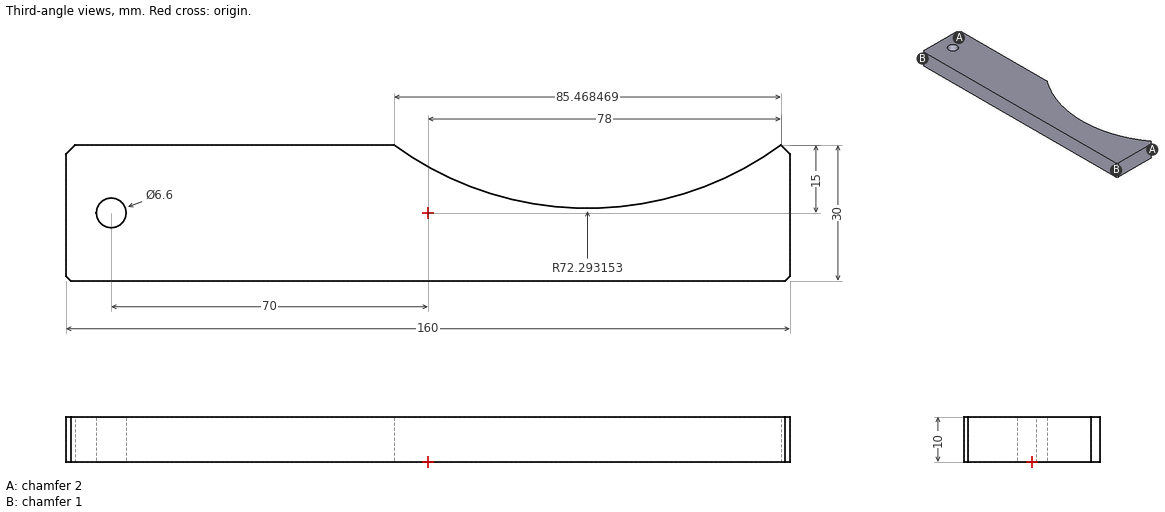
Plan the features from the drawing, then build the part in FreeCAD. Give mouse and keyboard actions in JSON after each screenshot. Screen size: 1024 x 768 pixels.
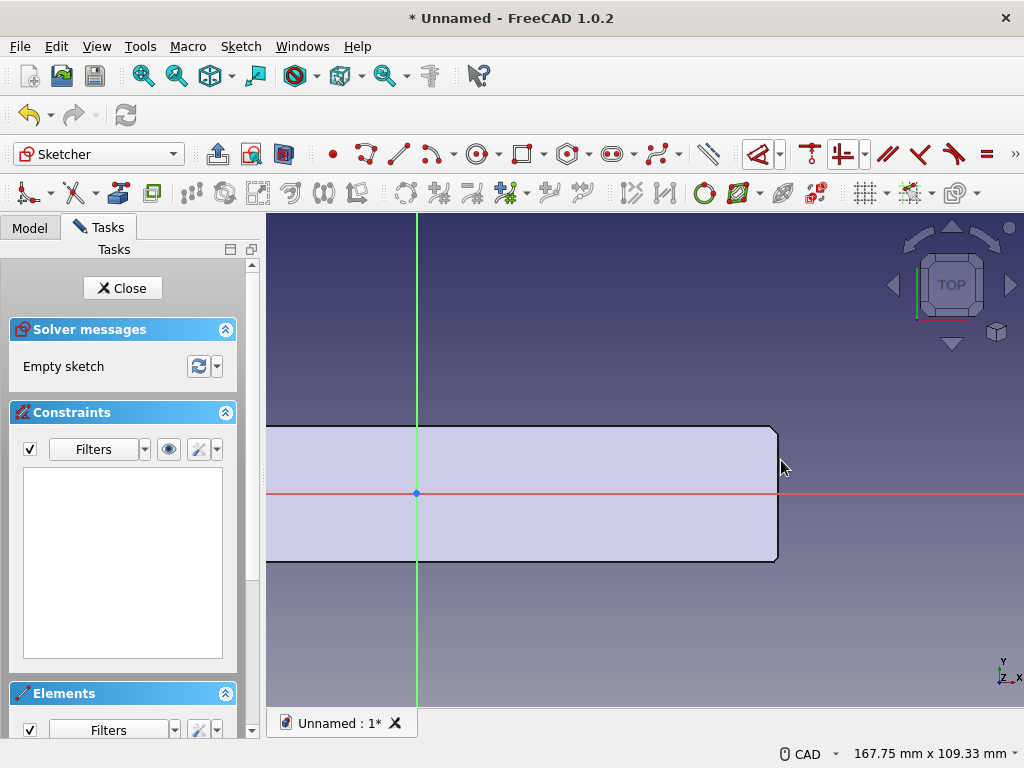
{"action": "left_click", "coordinate": [399, 154]}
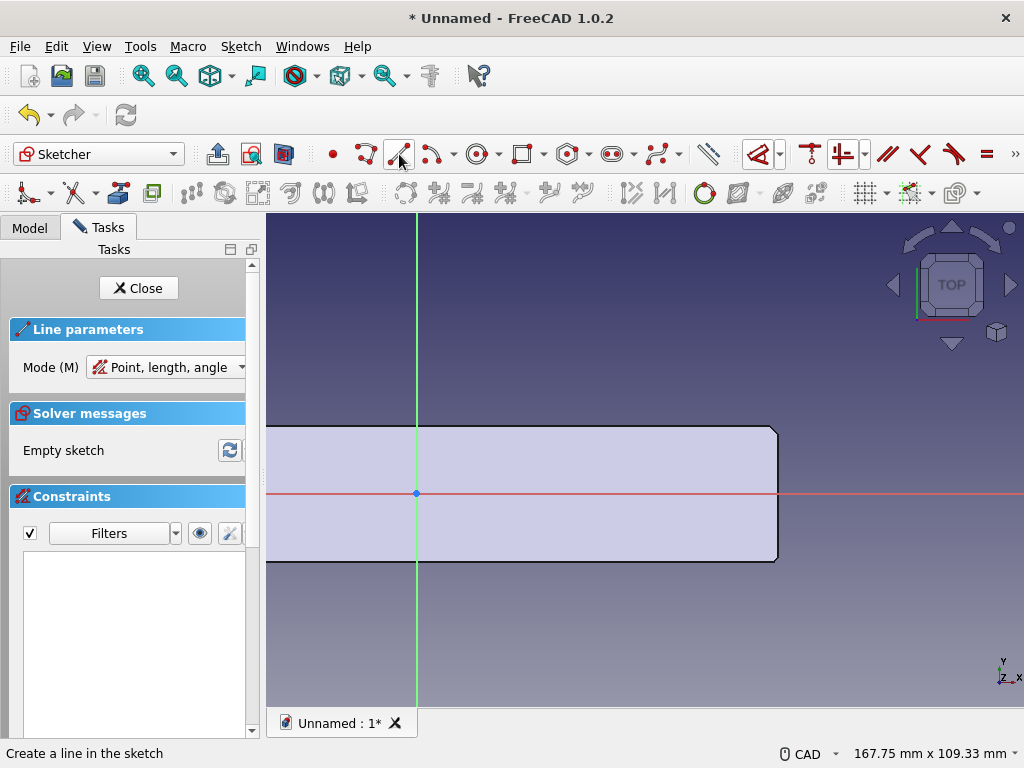
{"action": "left_click", "coordinate": [769, 426]}
{"action": "left_click", "coordinate": [383, 426]}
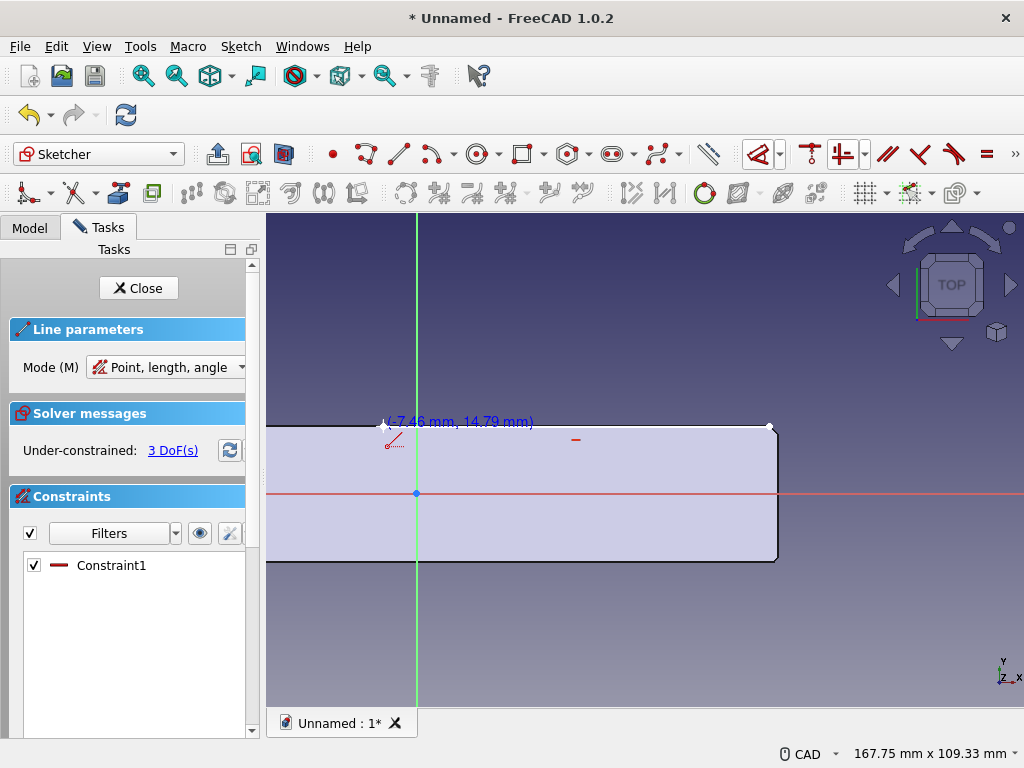
{"action": "key", "text": "g 3 a"}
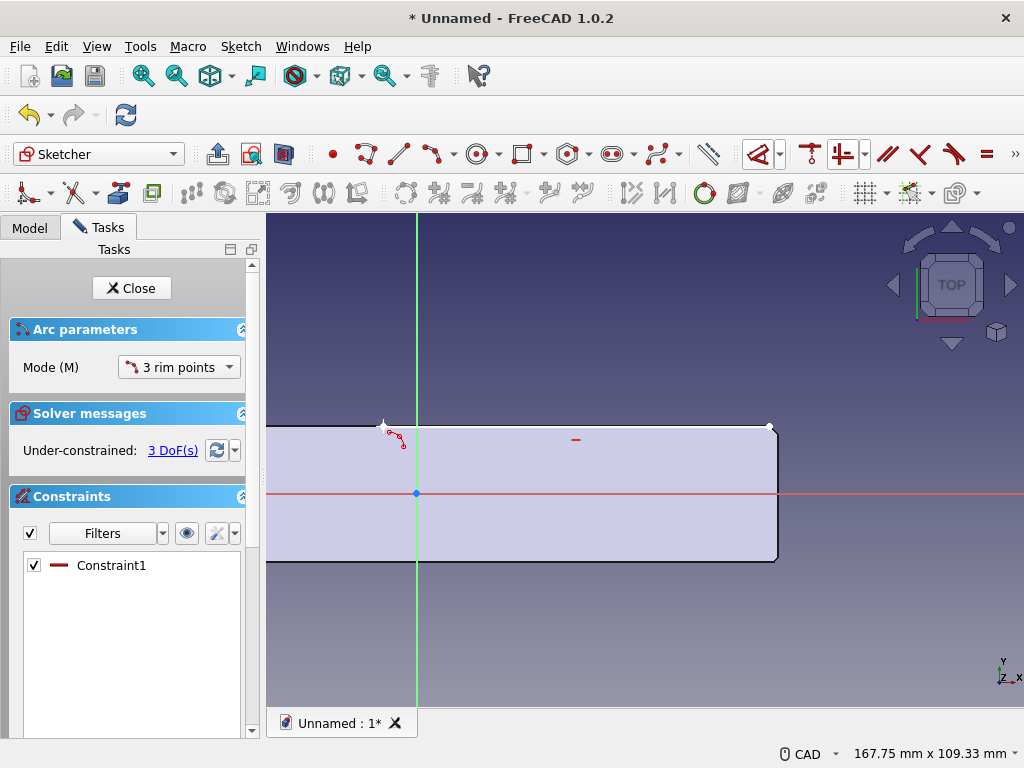
{"action": "left_click", "coordinate": [383, 427]}
{"action": "left_click", "coordinate": [769, 427]}
{"action": "left_click", "coordinate": [494, 479]}
{"action": "key", "text": "Escape"}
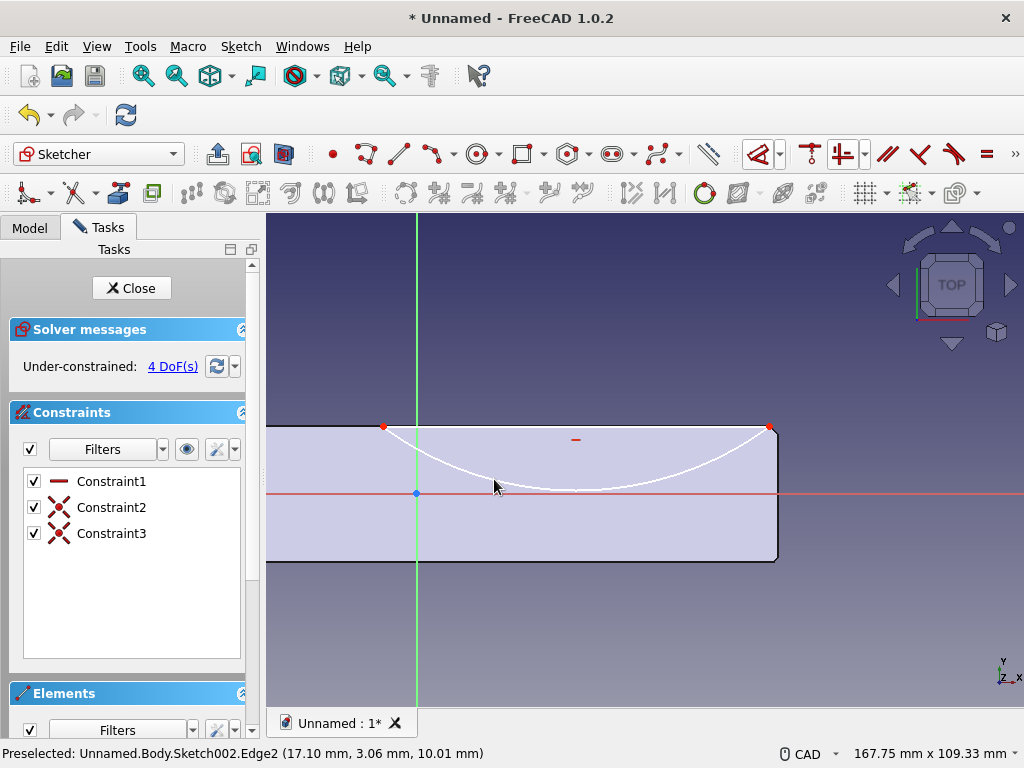
{"action": "left_click", "coordinate": [758, 154]}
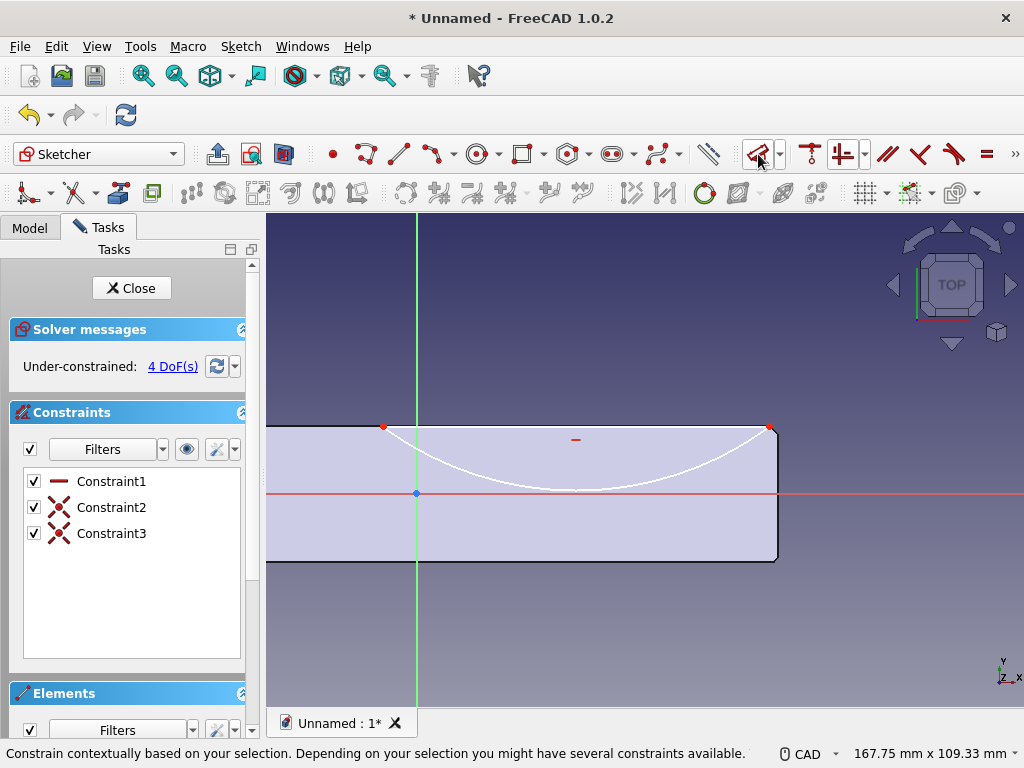
{"action": "left_click", "coordinate": [494, 480]}
{"action": "left_click", "coordinate": [486, 511]}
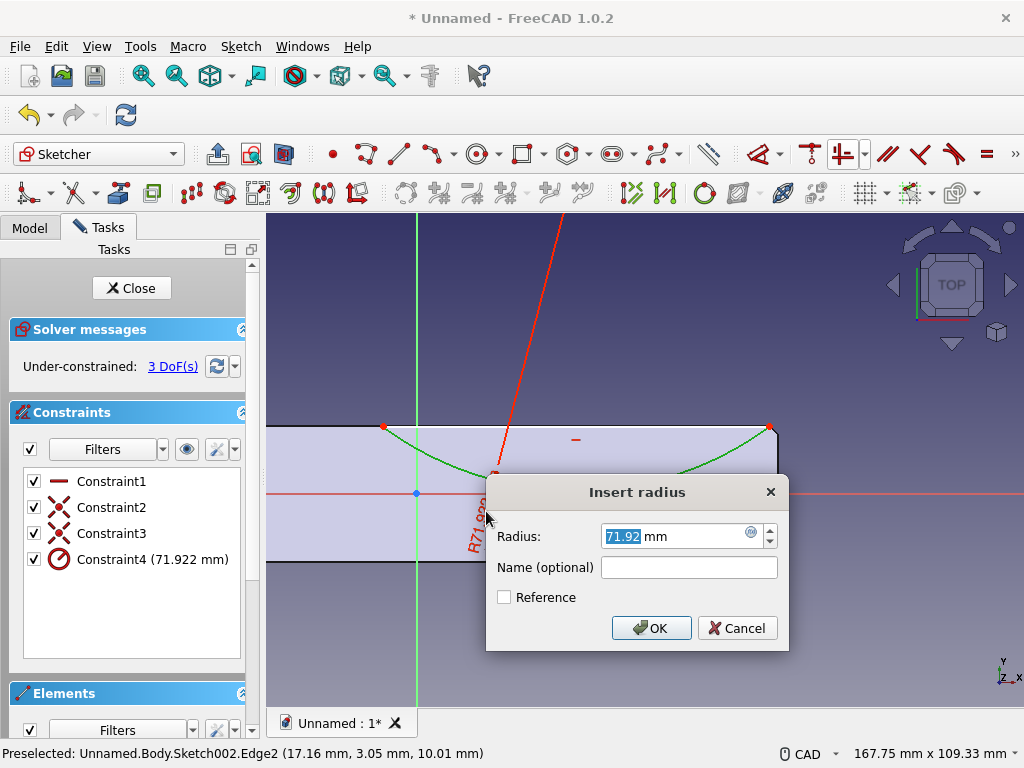
{"action": "type", "text": "72.293153"}
{"action": "key", "text": "Return"}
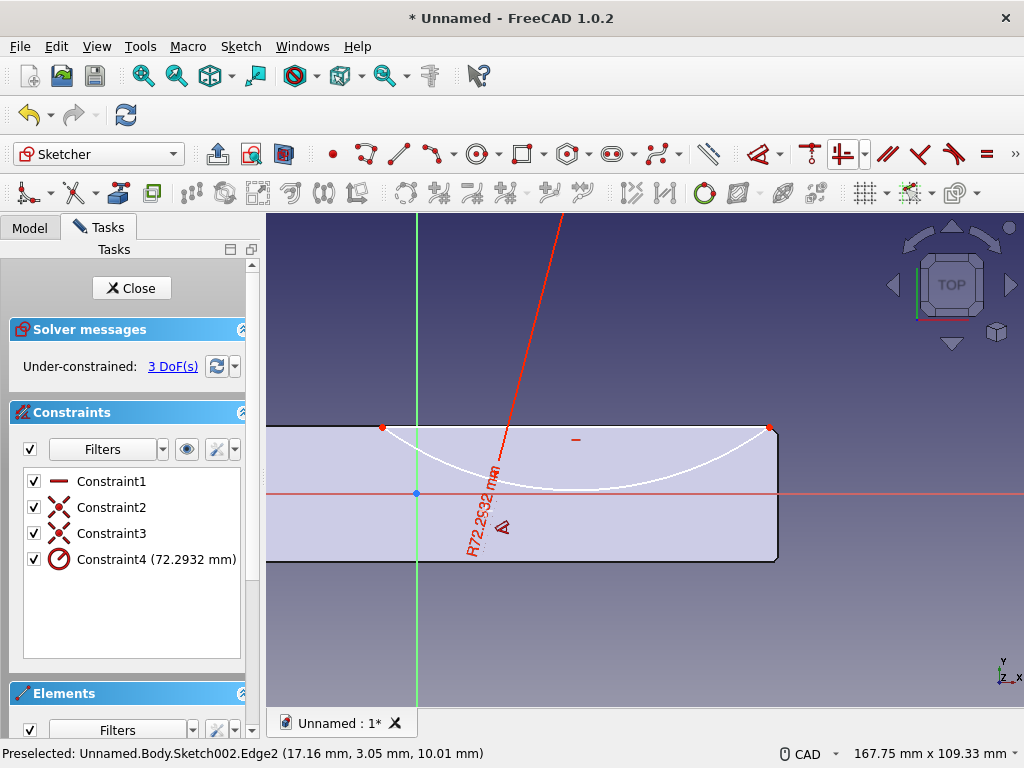
{"action": "left_click", "coordinate": [769, 427]}
{"action": "left_click", "coordinate": [593, 528]}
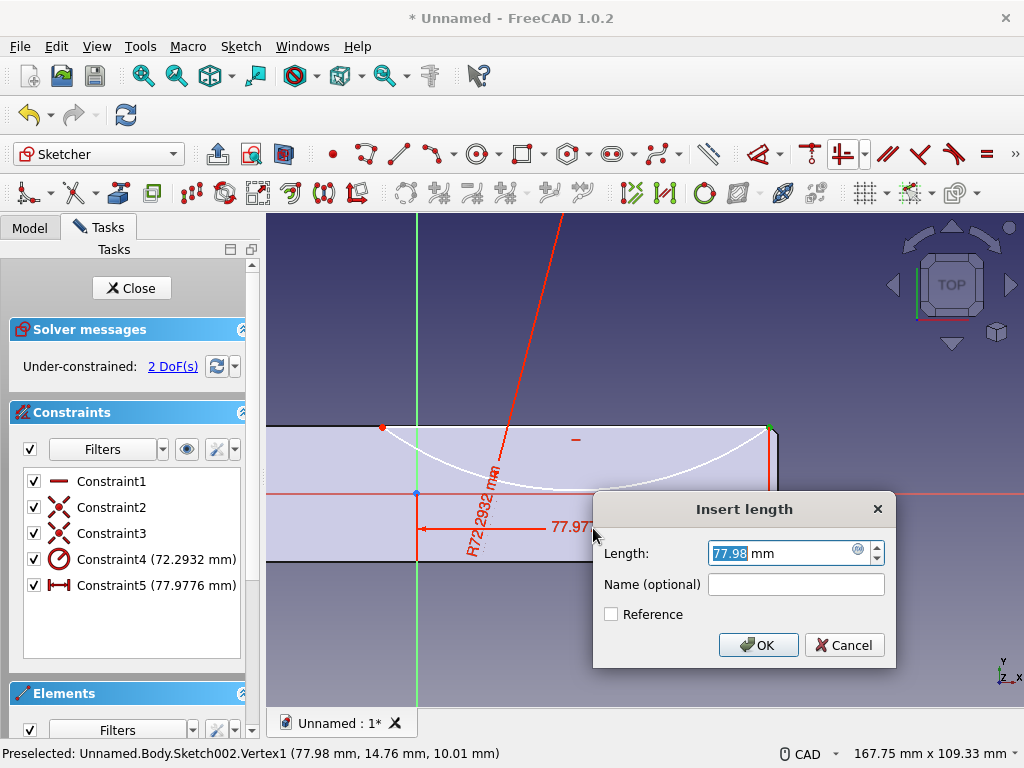
{"action": "type", "text": "78"}
{"action": "key", "text": "Return"}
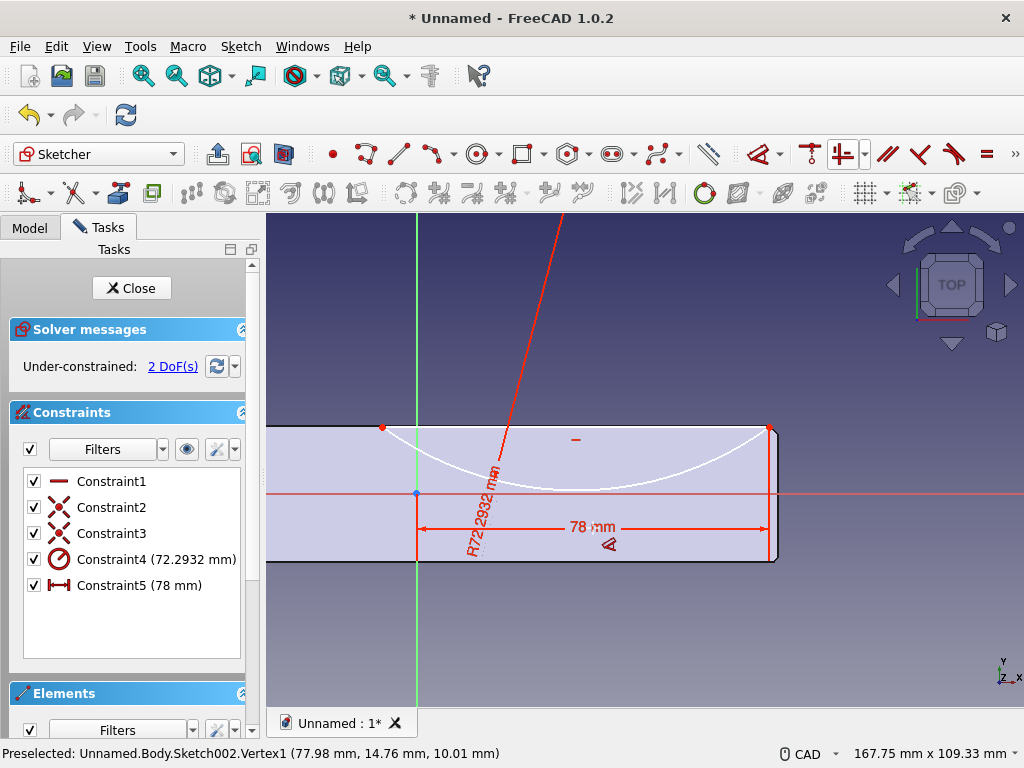
{"action": "left_click", "coordinate": [769, 427]}
{"action": "left_click", "coordinate": [803, 461]}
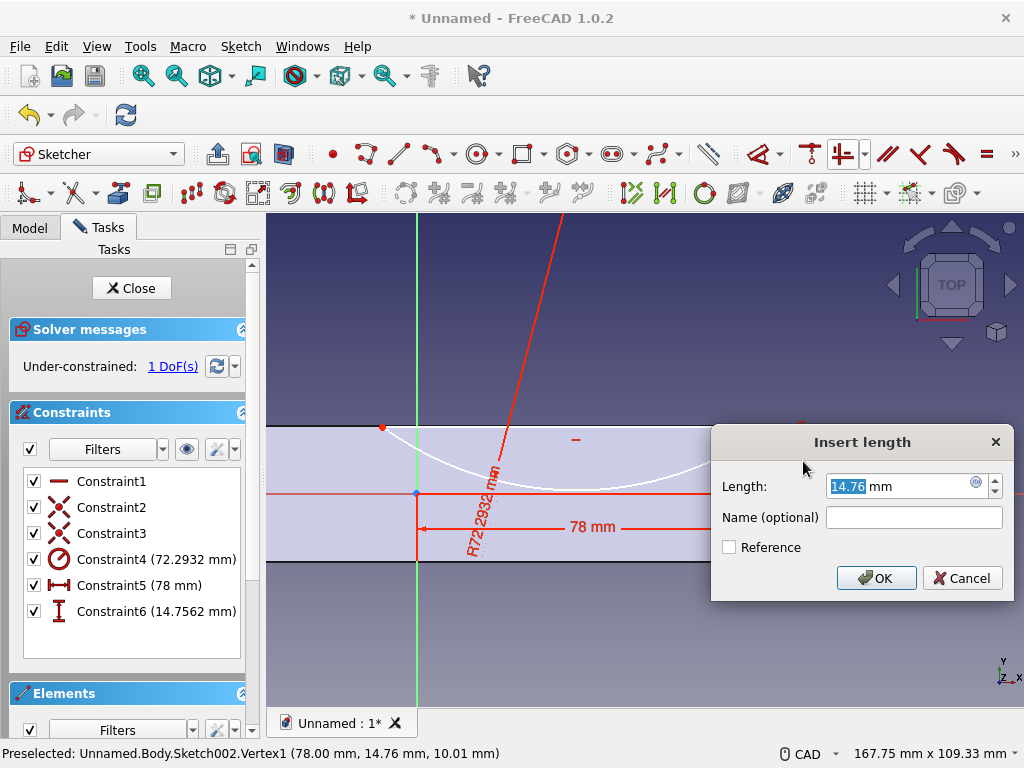
{"action": "type", "text": "15"}
{"action": "key", "text": "Return"}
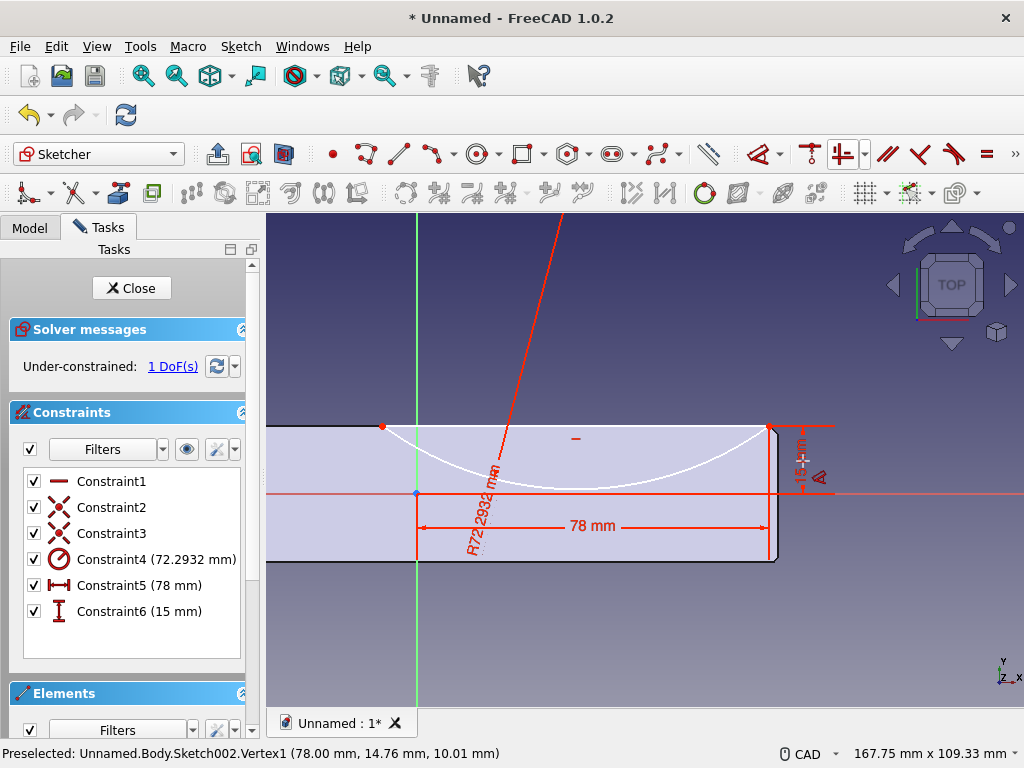
{"action": "left_click", "coordinate": [653, 426]}
{"action": "left_click", "coordinate": [576, 392]}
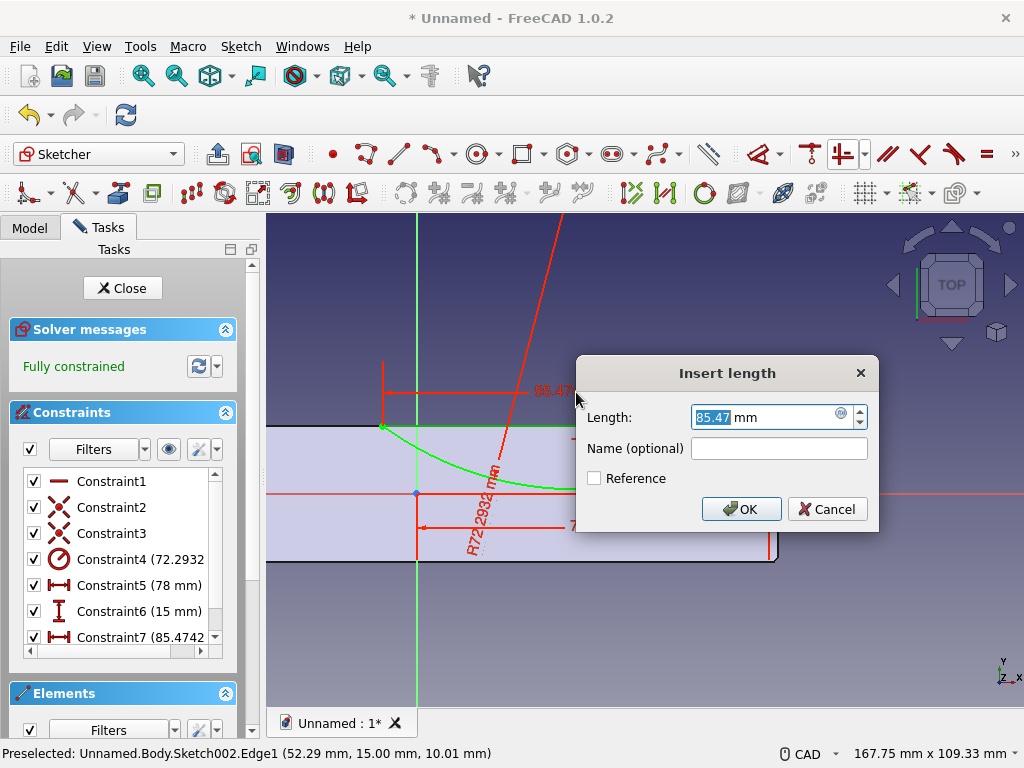
{"action": "type", "text": "85.468469"}
{"action": "key", "text": "Return"}
{"action": "key", "text": "Escape"}